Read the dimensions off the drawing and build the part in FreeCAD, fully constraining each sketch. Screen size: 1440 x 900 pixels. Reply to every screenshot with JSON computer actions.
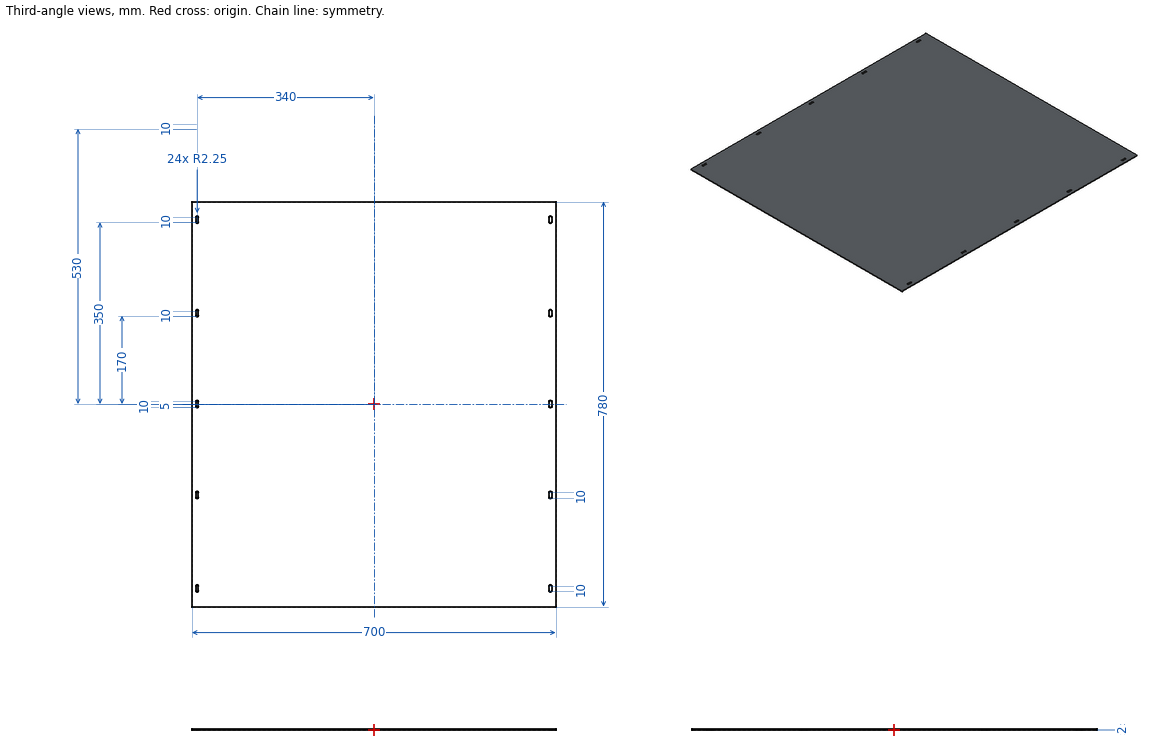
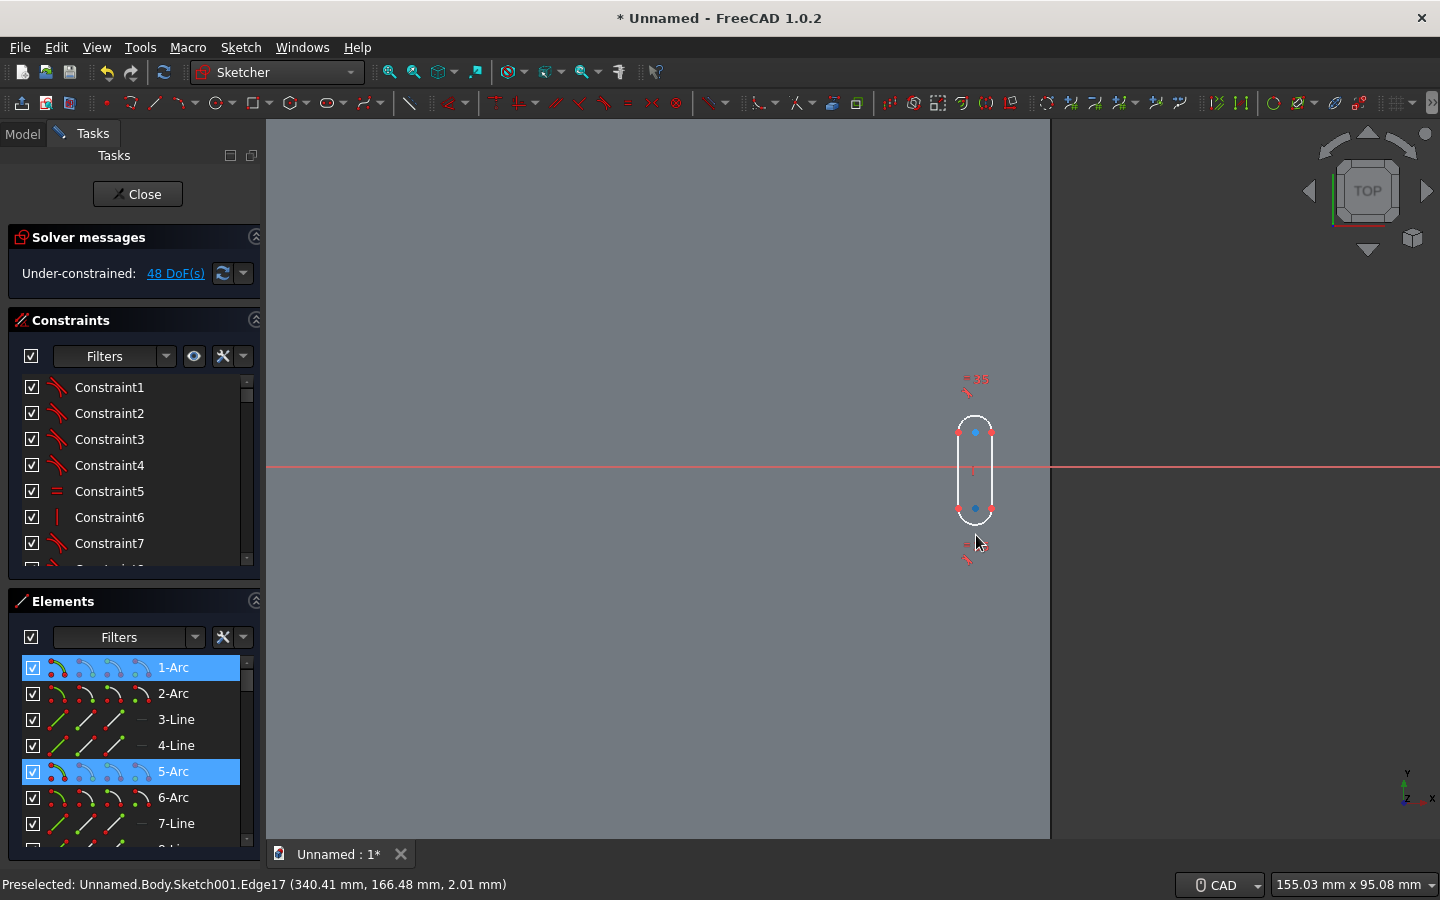
{"action": "left_click", "coordinate": [965, 522]}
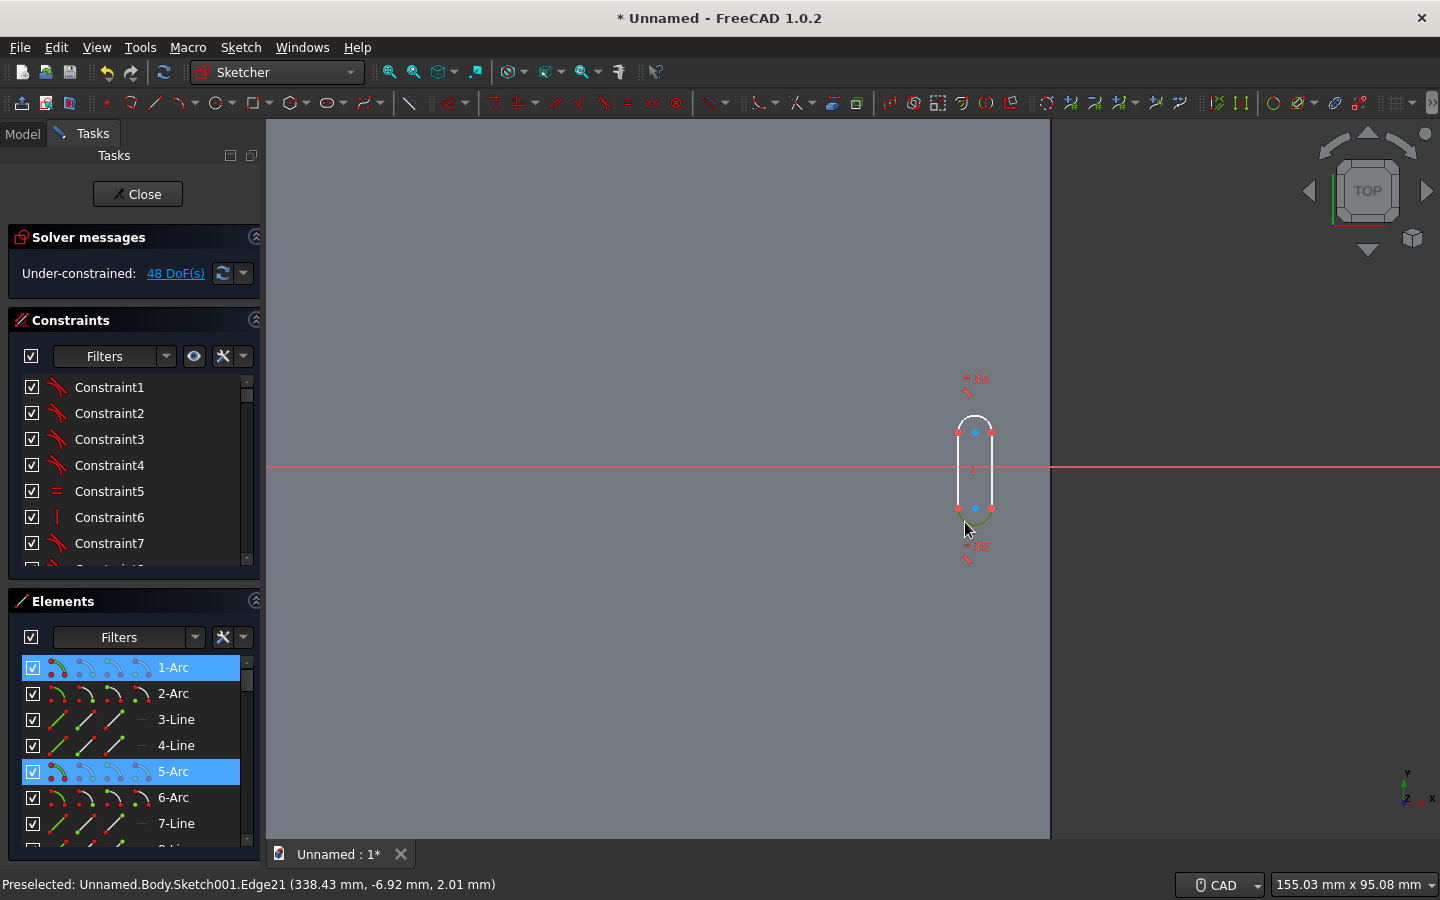
{"action": "scroll", "coordinate": [976, 535], "scroll_direction": "down", "scroll_amount": 13}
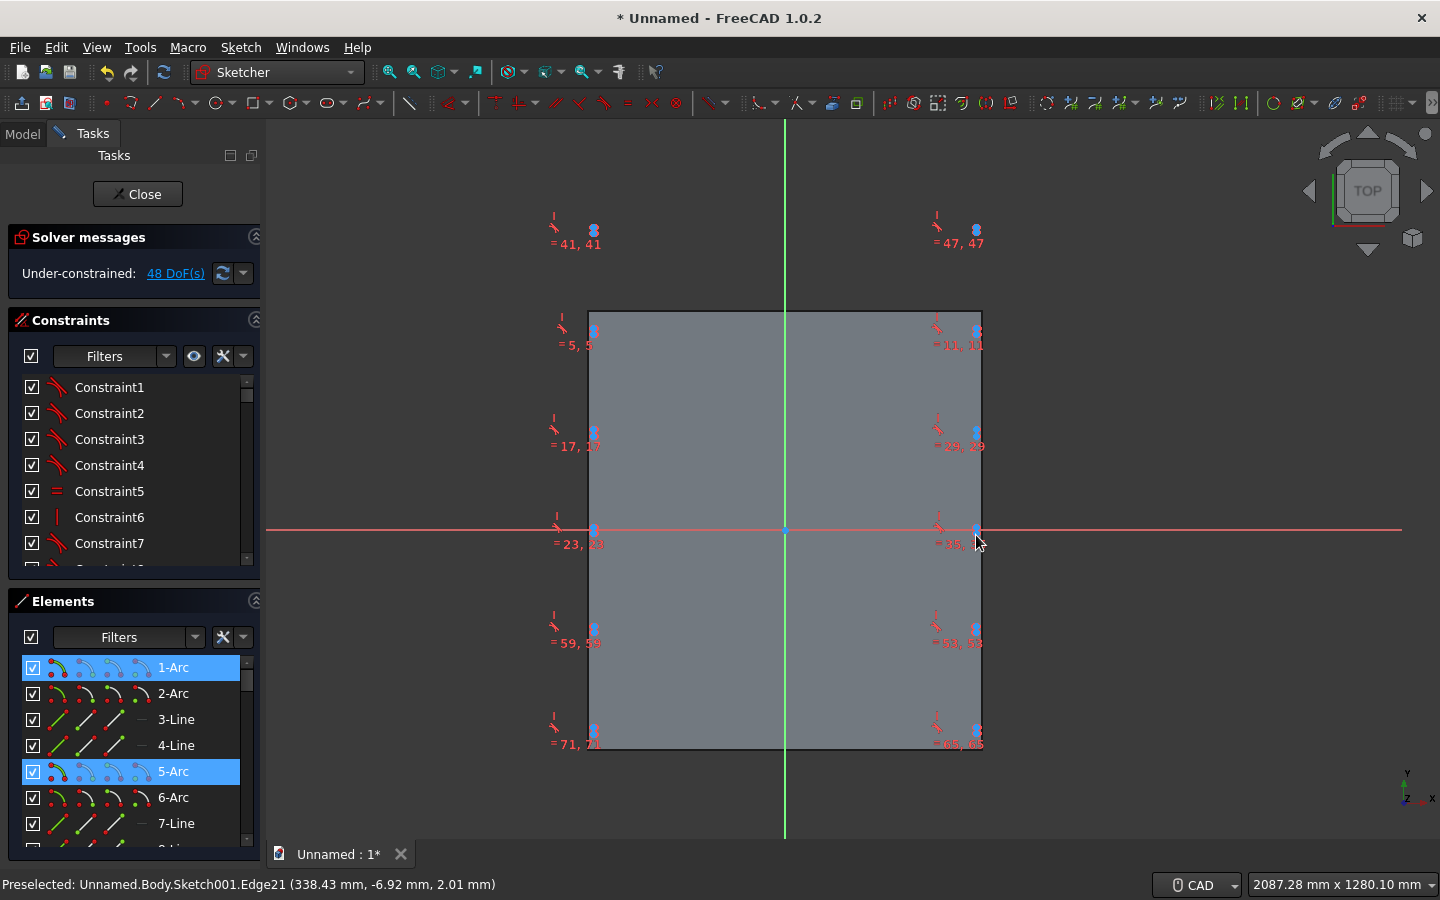
{"action": "scroll", "coordinate": [593, 234], "scroll_direction": "up", "scroll_amount": 13}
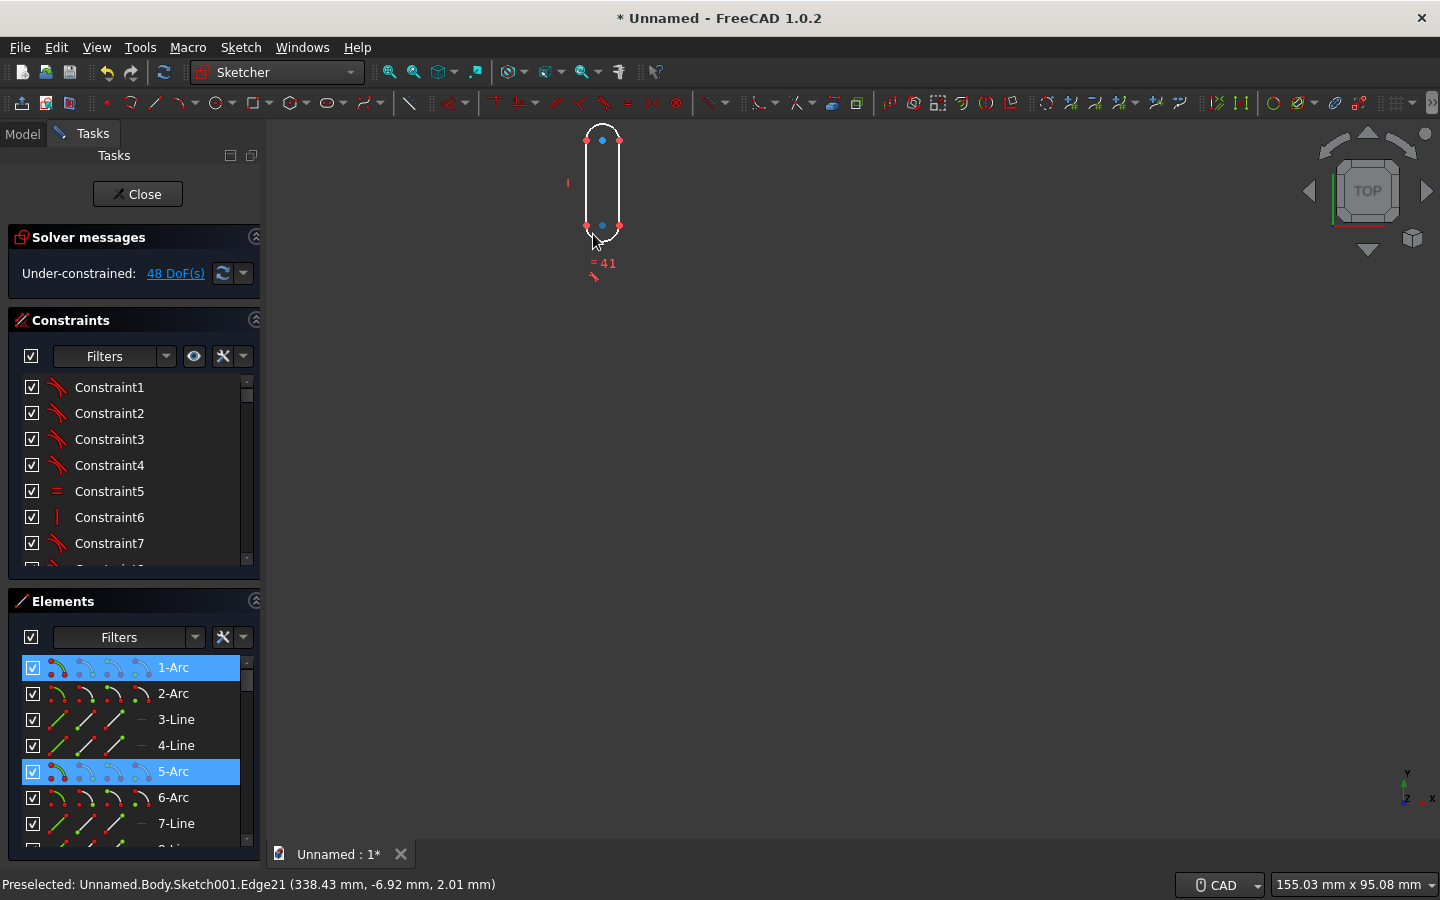
{"action": "left_click", "coordinate": [593, 238]}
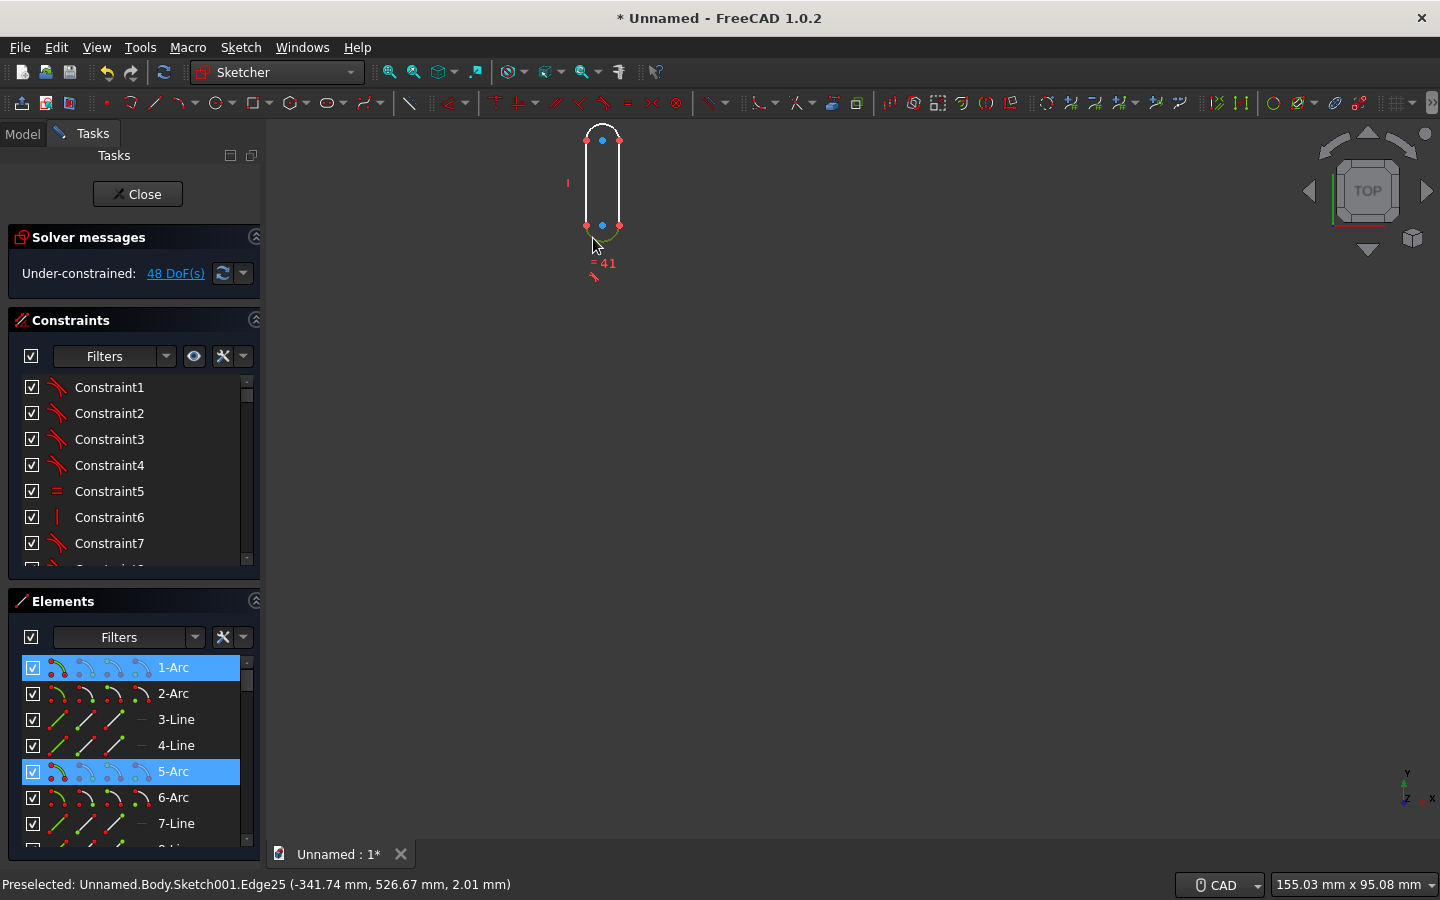
{"action": "scroll", "coordinate": [592, 233], "scroll_direction": "down", "scroll_amount": 13}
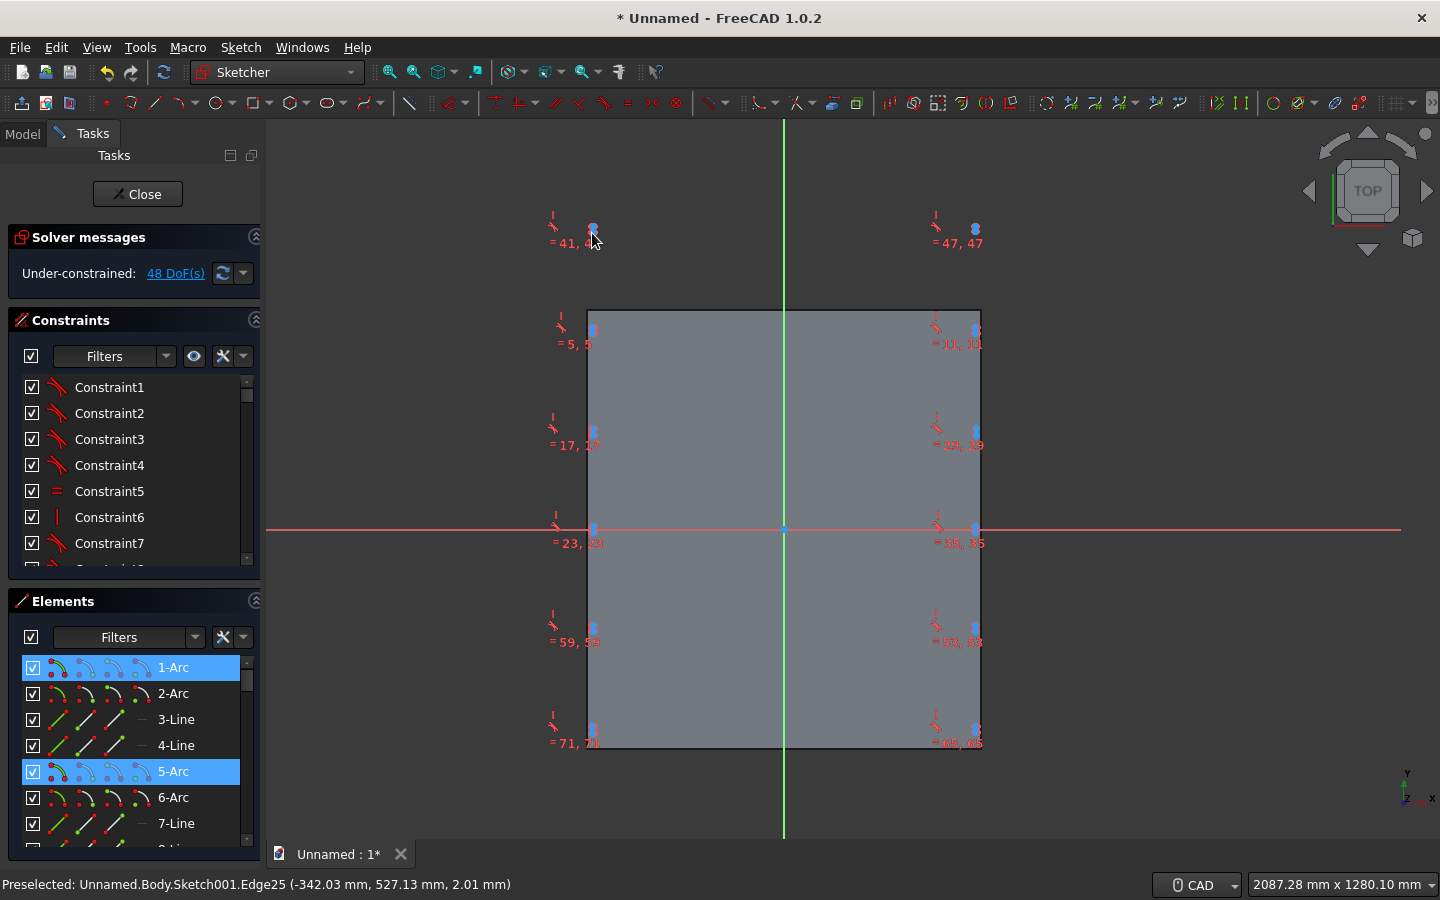
{"action": "scroll", "coordinate": [975, 233], "scroll_direction": "up", "scroll_amount": 14}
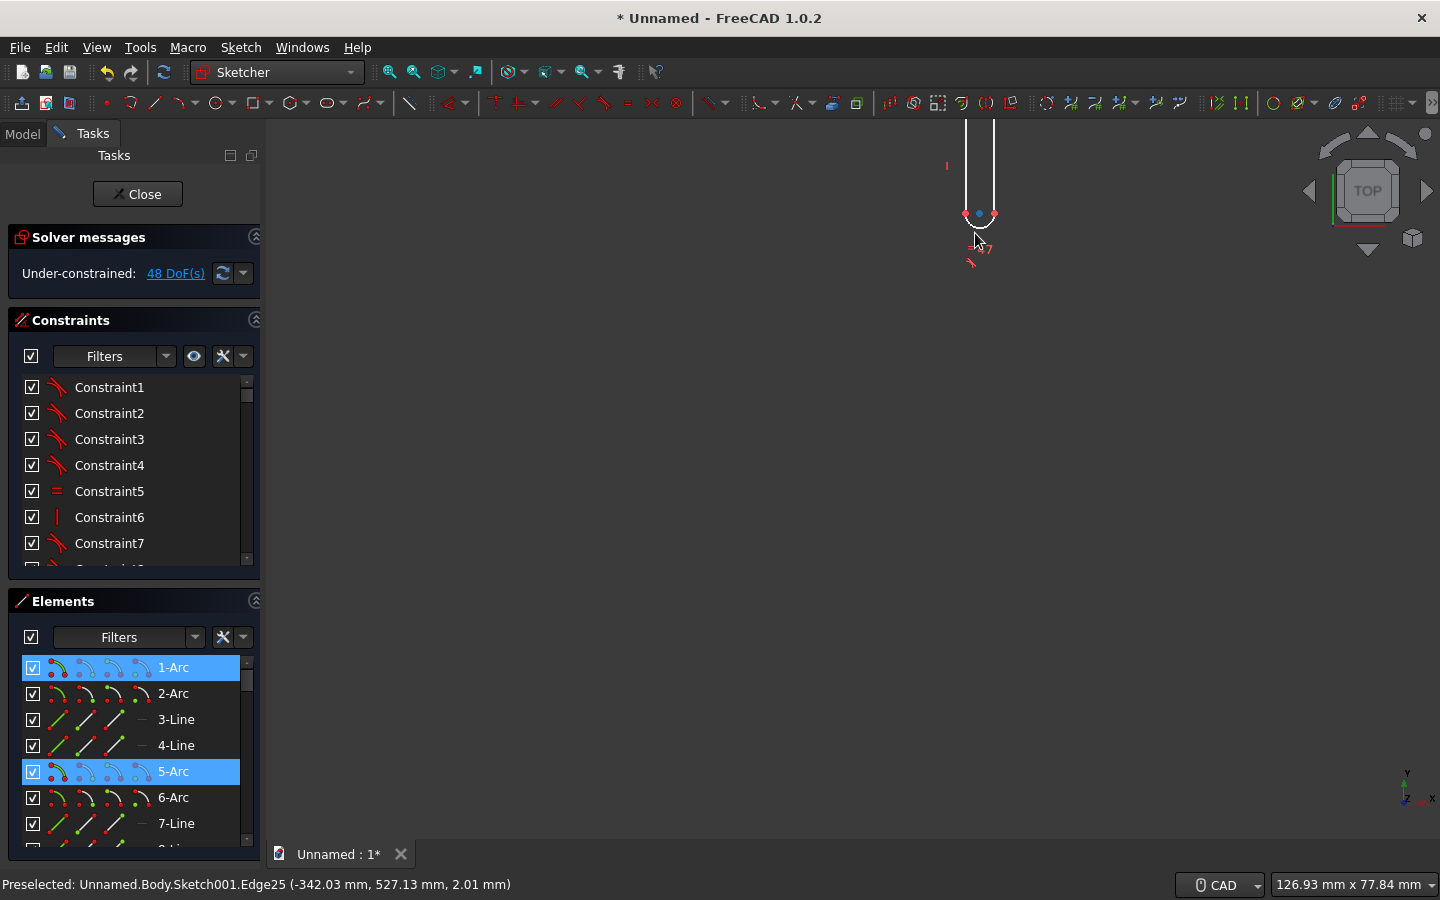
{"action": "left_click", "coordinate": [972, 225]}